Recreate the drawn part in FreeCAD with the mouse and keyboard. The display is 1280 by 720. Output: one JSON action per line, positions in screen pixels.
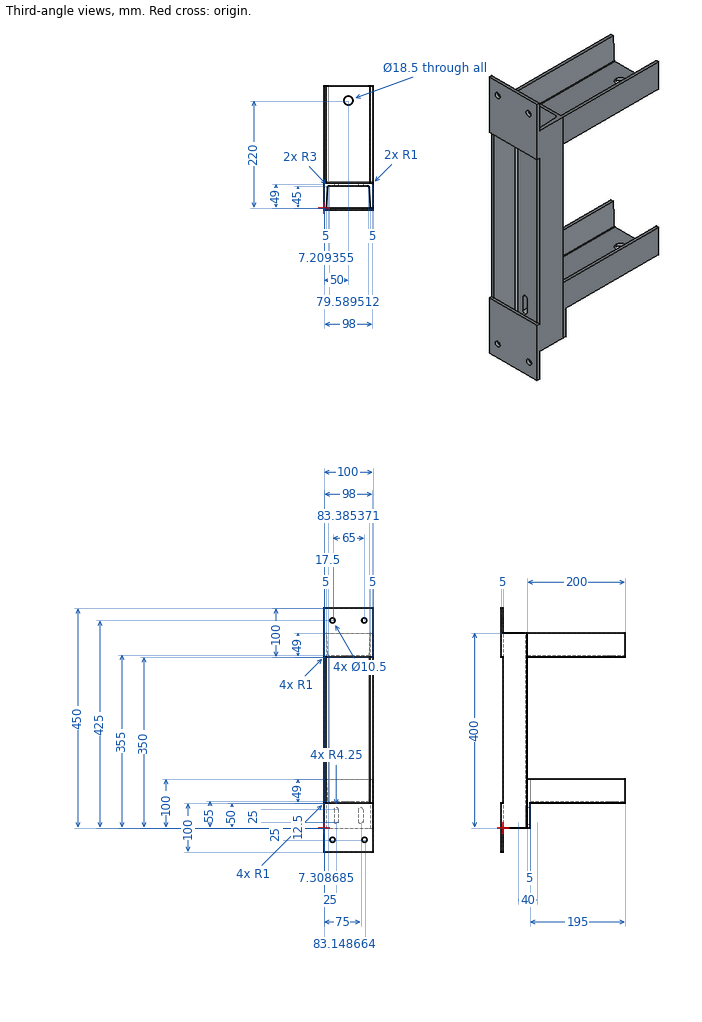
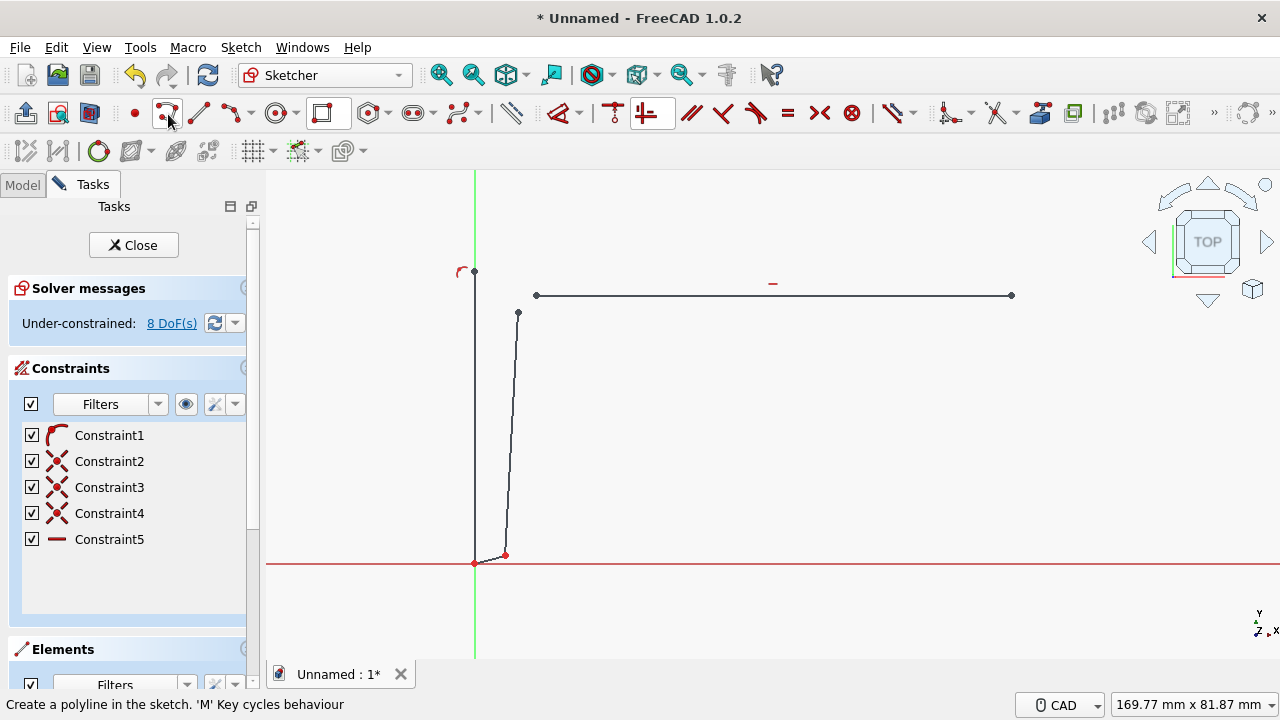
{"action": "left_click", "coordinate": [1029, 312]}
{"action": "left_click", "coordinate": [1042, 564]}
{"action": "left_click", "coordinate": [1072, 555]}
{"action": "left_click", "coordinate": [1072, 271]}
{"action": "right_click", "coordinate": [1072, 271]}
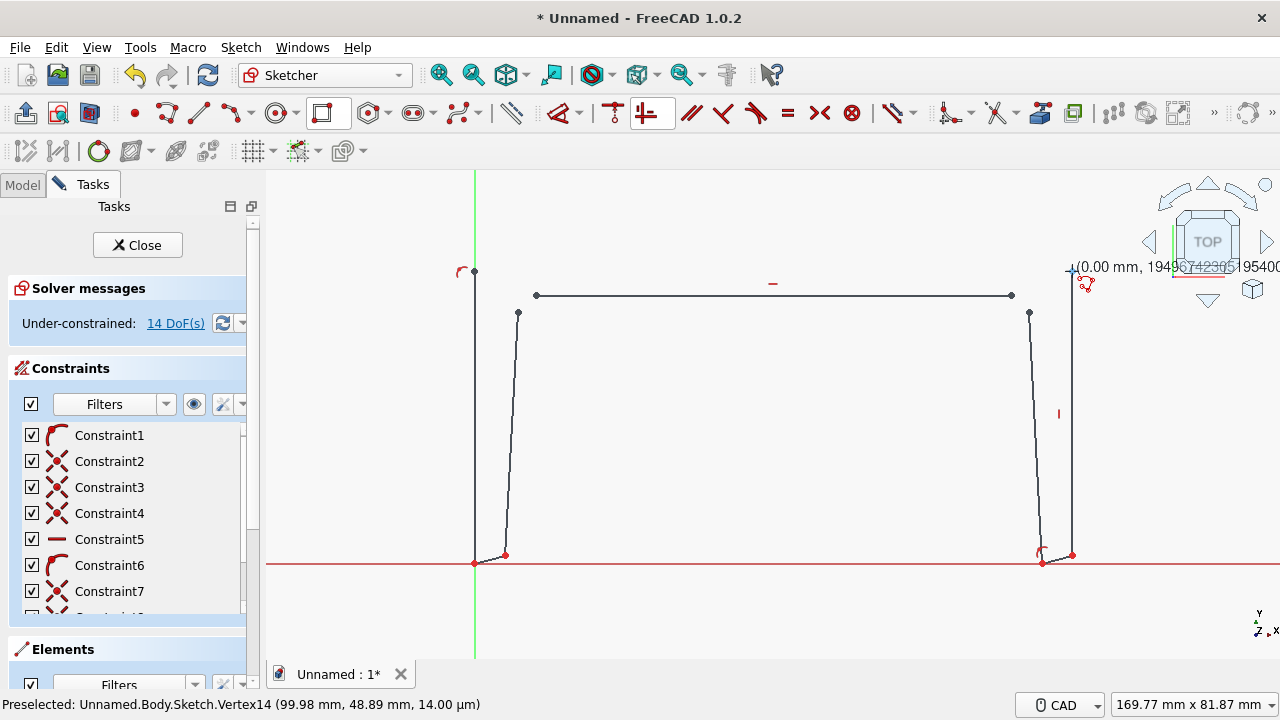
{"action": "left_click", "coordinate": [200, 114]}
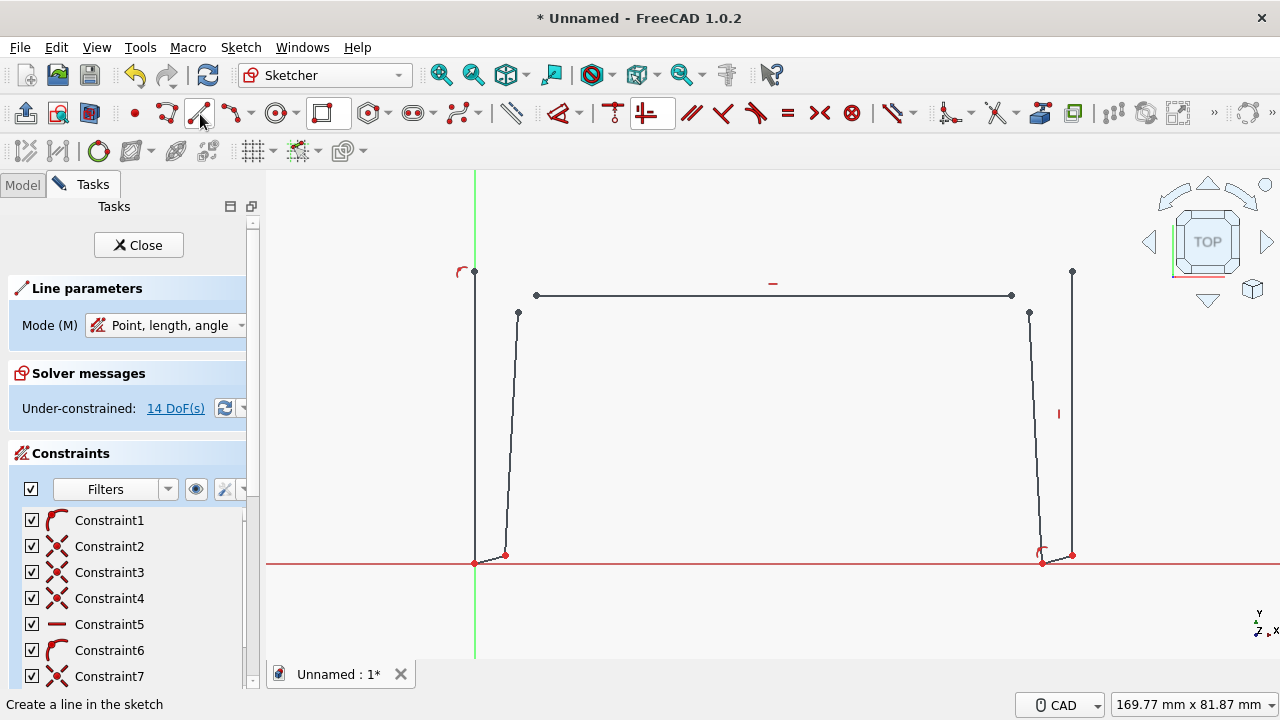
{"action": "scroll", "coordinate": [1066, 265], "scroll_direction": "up", "scroll_amount": 4}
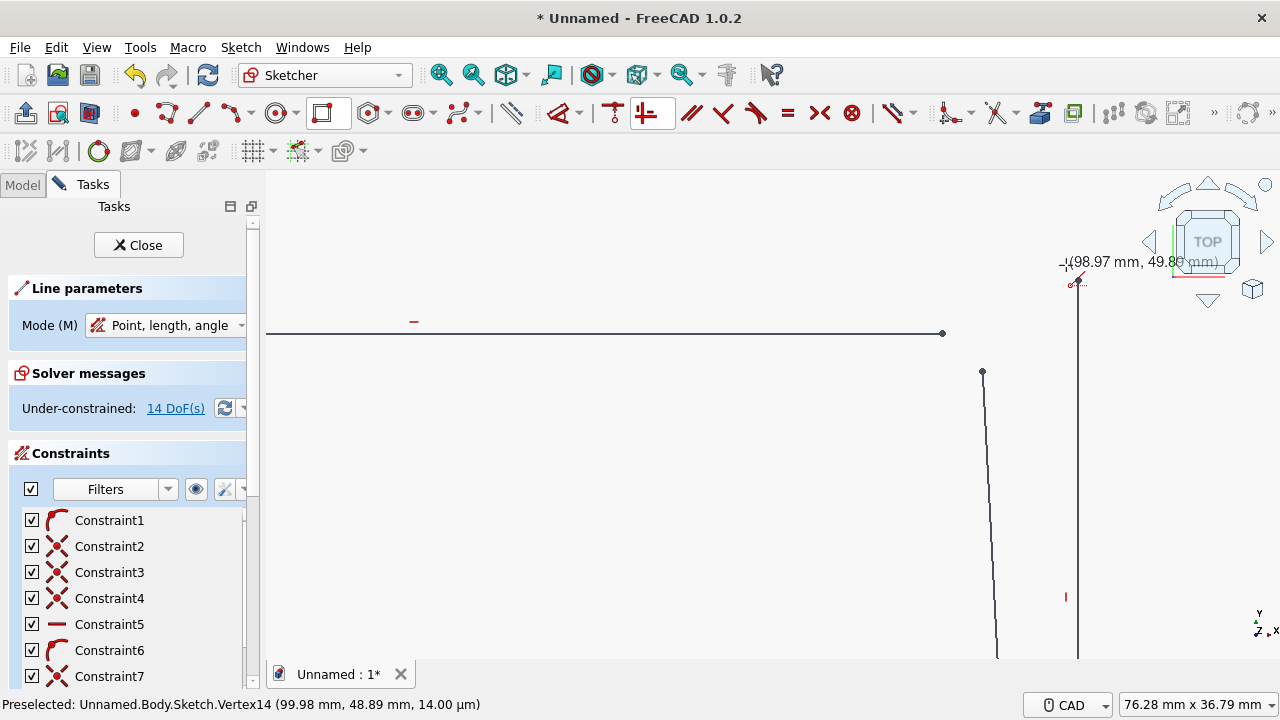
{"action": "left_click", "coordinate": [1065, 266]}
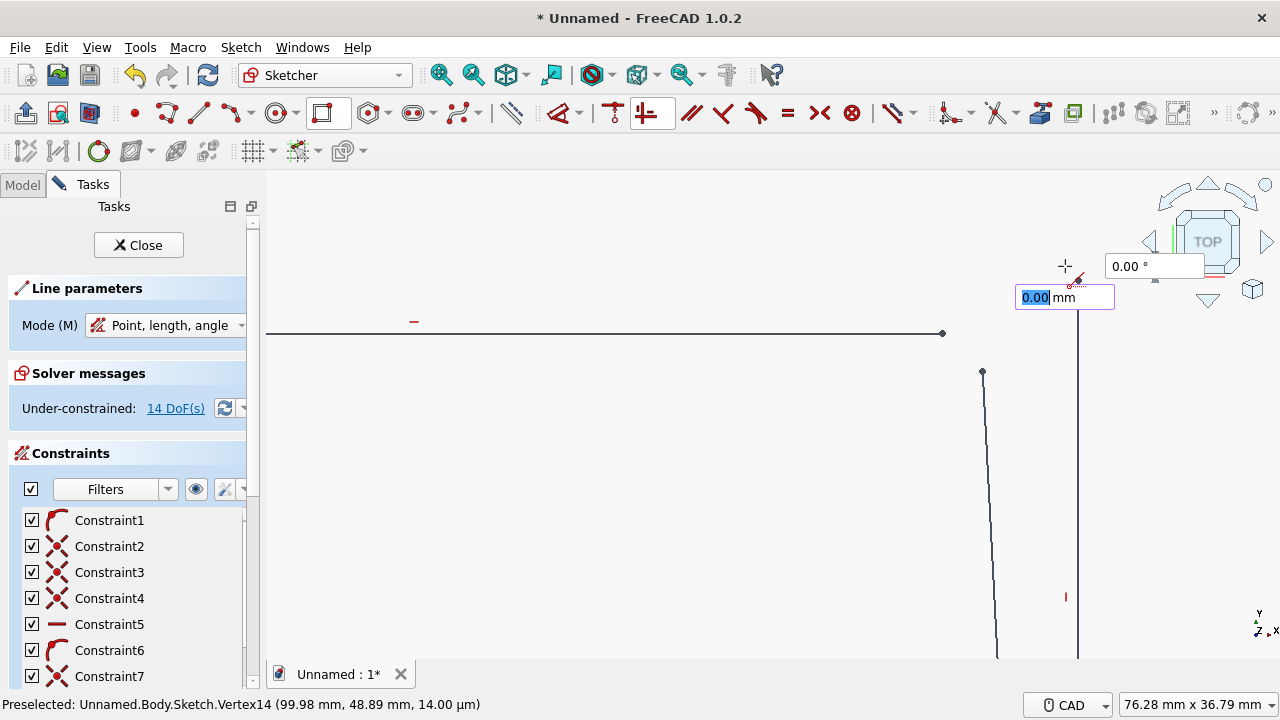
{"action": "scroll", "coordinate": [942, 265], "scroll_direction": "down", "scroll_amount": 4}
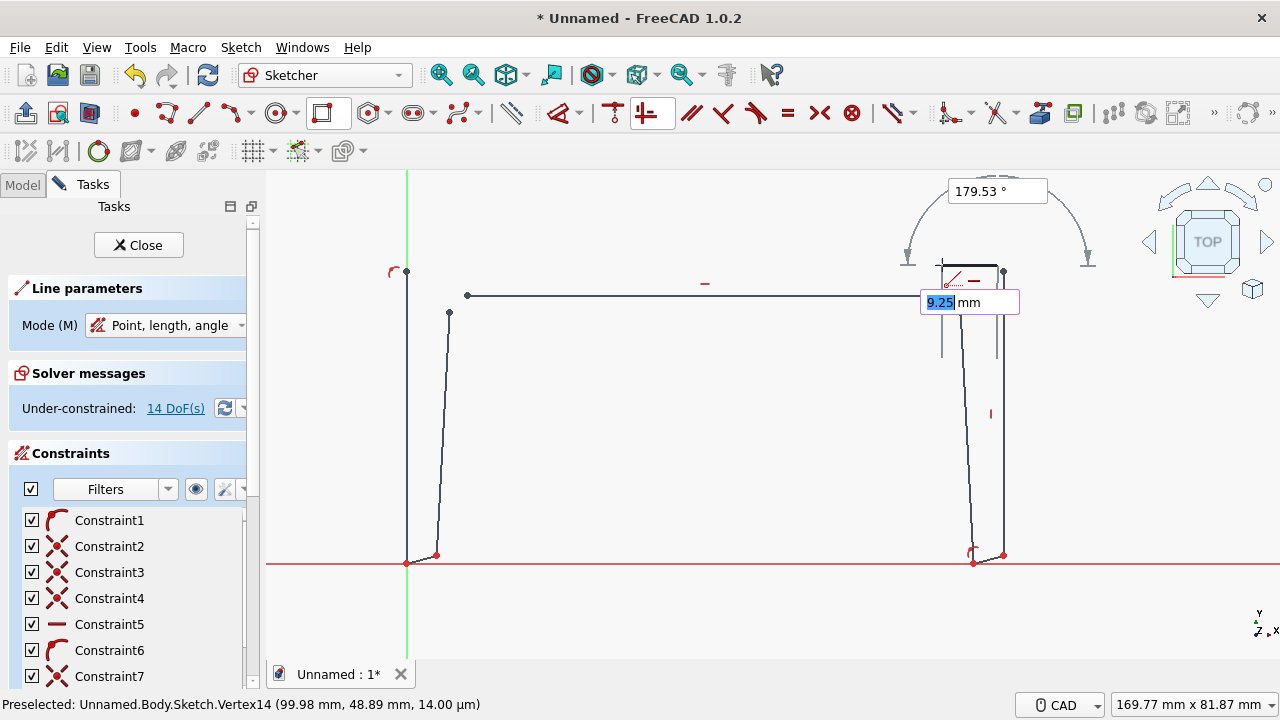
{"action": "scroll", "coordinate": [412, 265], "scroll_direction": "up", "scroll_amount": 5}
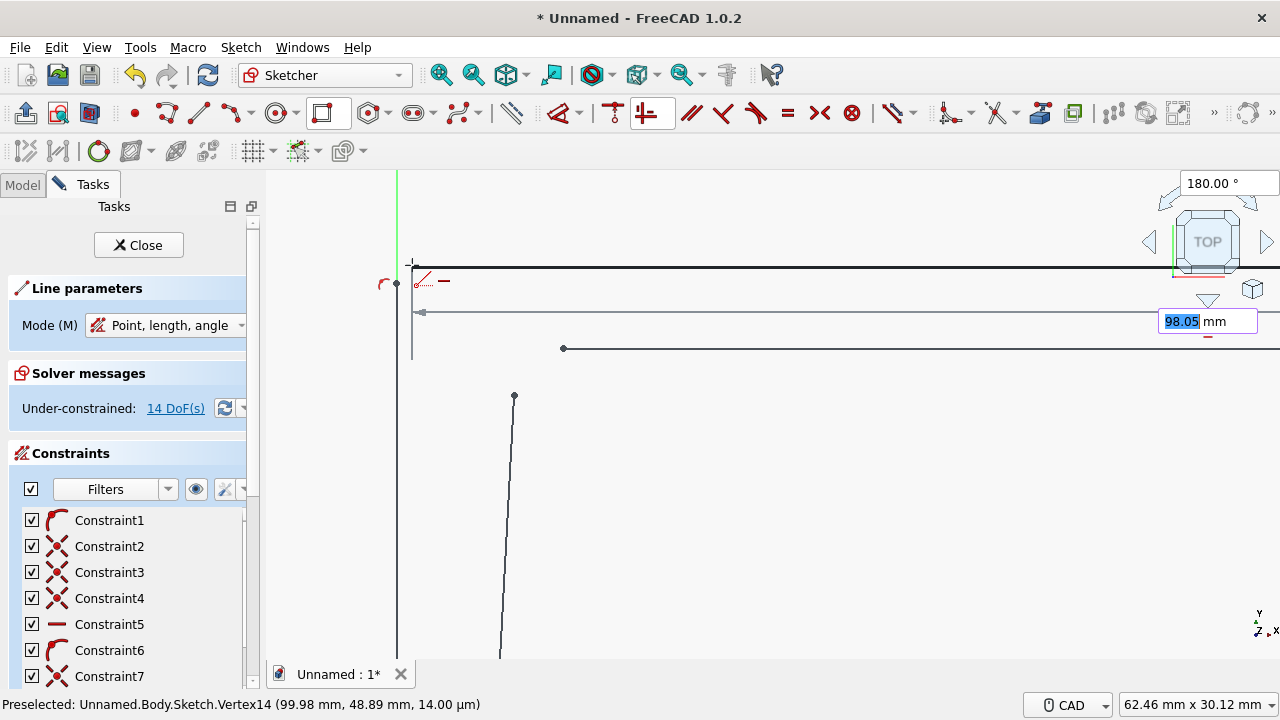
{"action": "left_click", "coordinate": [413, 266]}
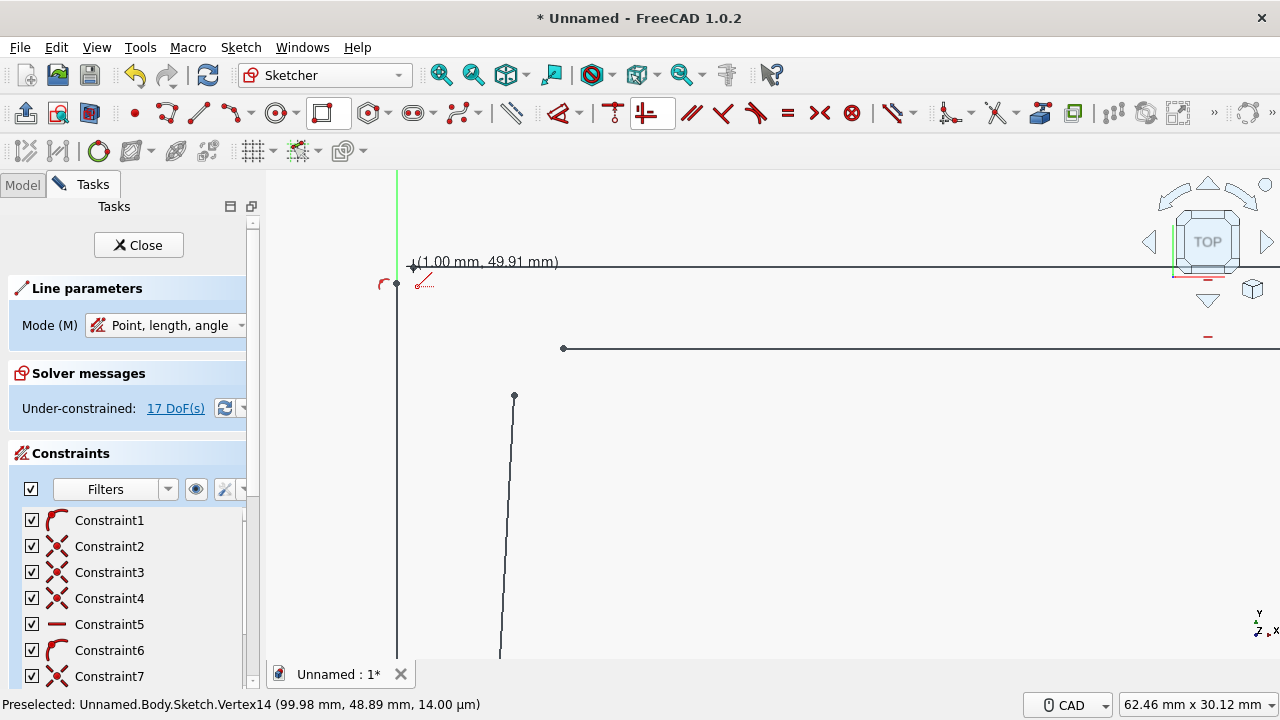
{"action": "left_click", "coordinate": [232, 114]}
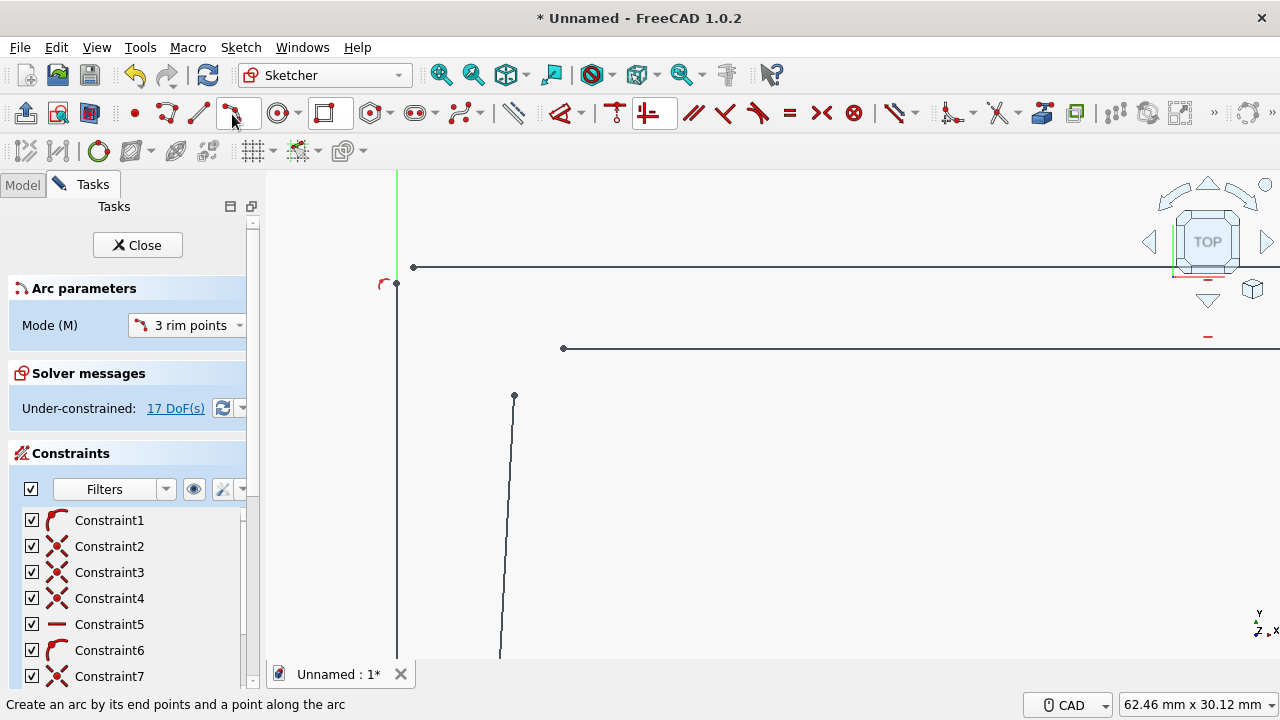
{"action": "left_click", "coordinate": [514, 395]}
{"action": "left_click", "coordinate": [563, 349]}
{"action": "left_click", "coordinate": [529, 360]}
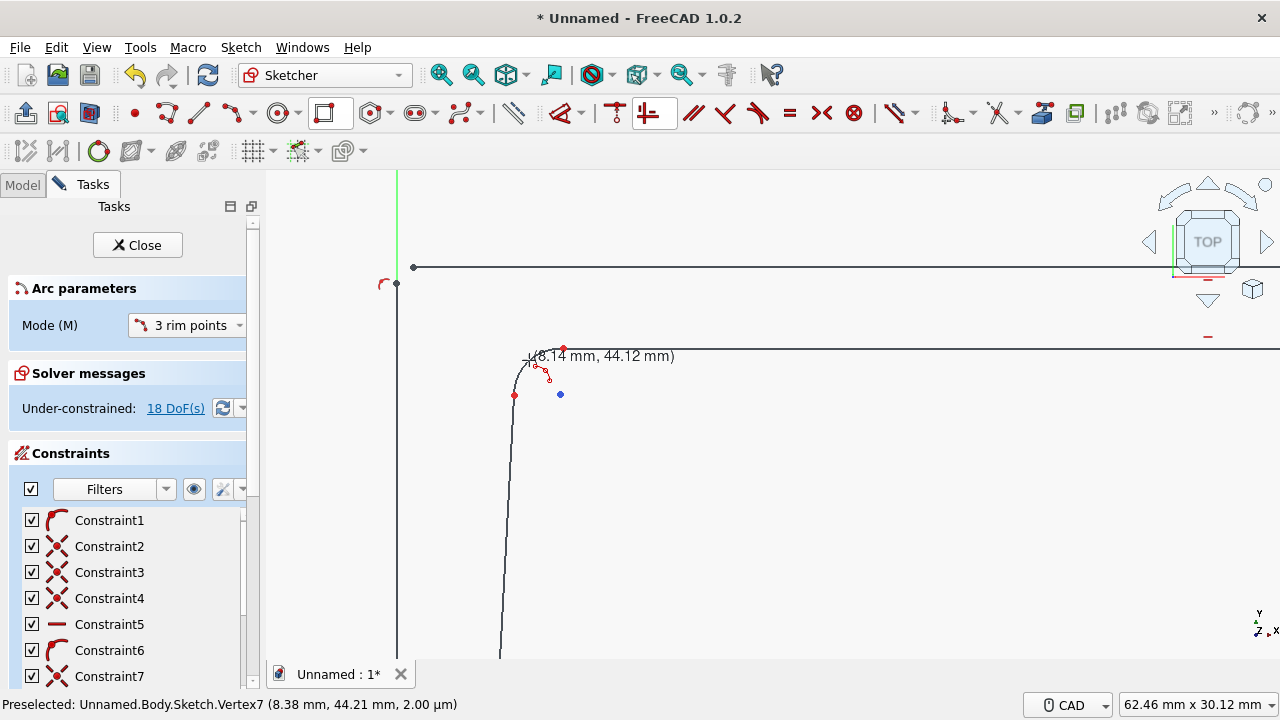
{"action": "scroll", "coordinate": [411, 265], "scroll_direction": "down", "scroll_amount": 5}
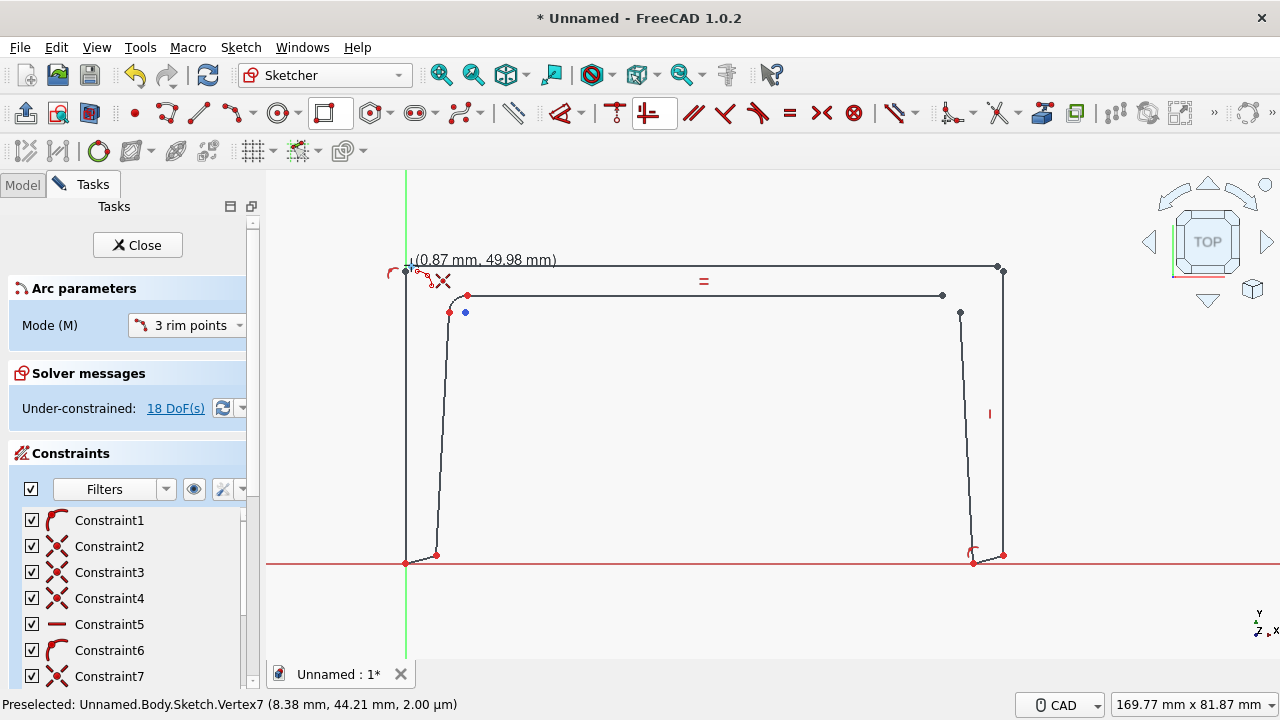
{"action": "left_click", "coordinate": [942, 296]}
{"action": "left_click", "coordinate": [960, 313]}